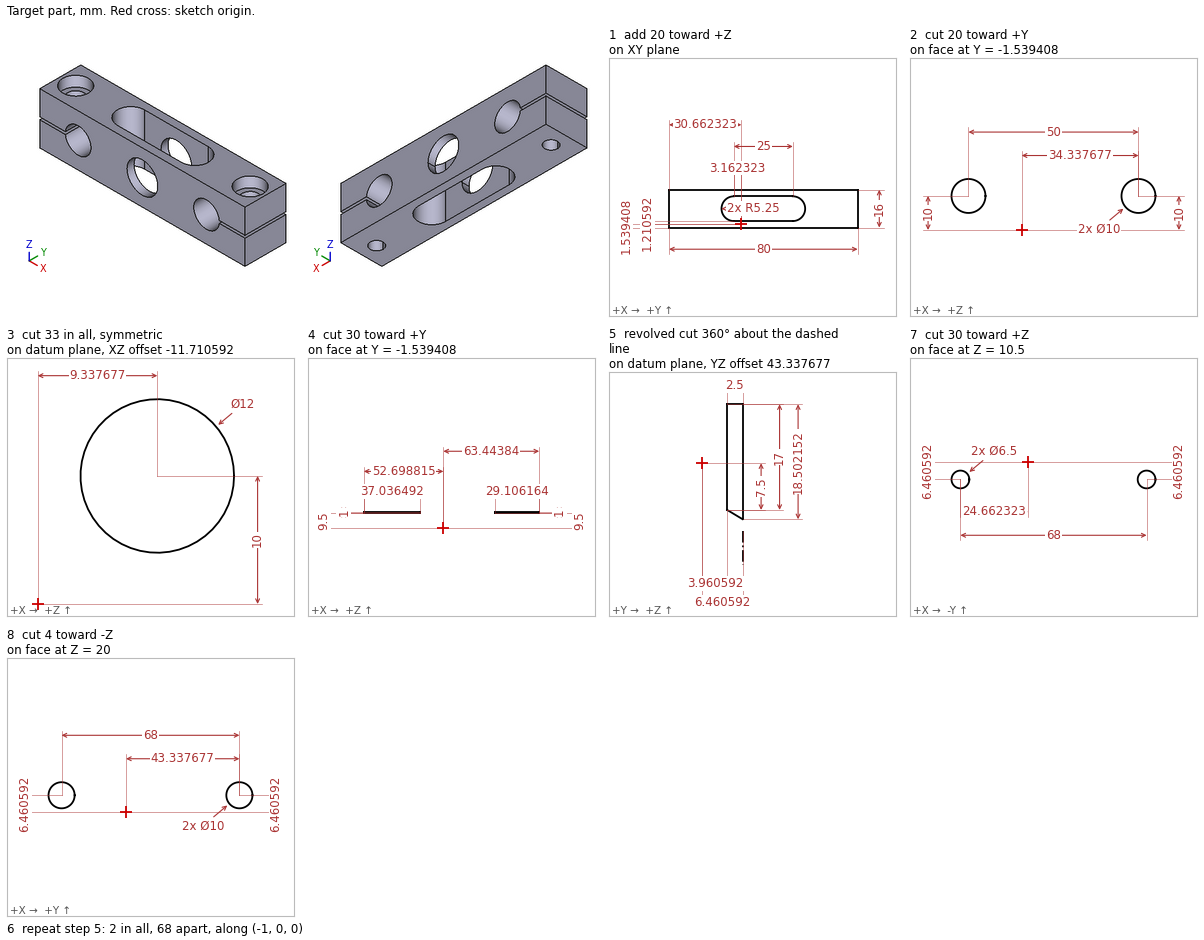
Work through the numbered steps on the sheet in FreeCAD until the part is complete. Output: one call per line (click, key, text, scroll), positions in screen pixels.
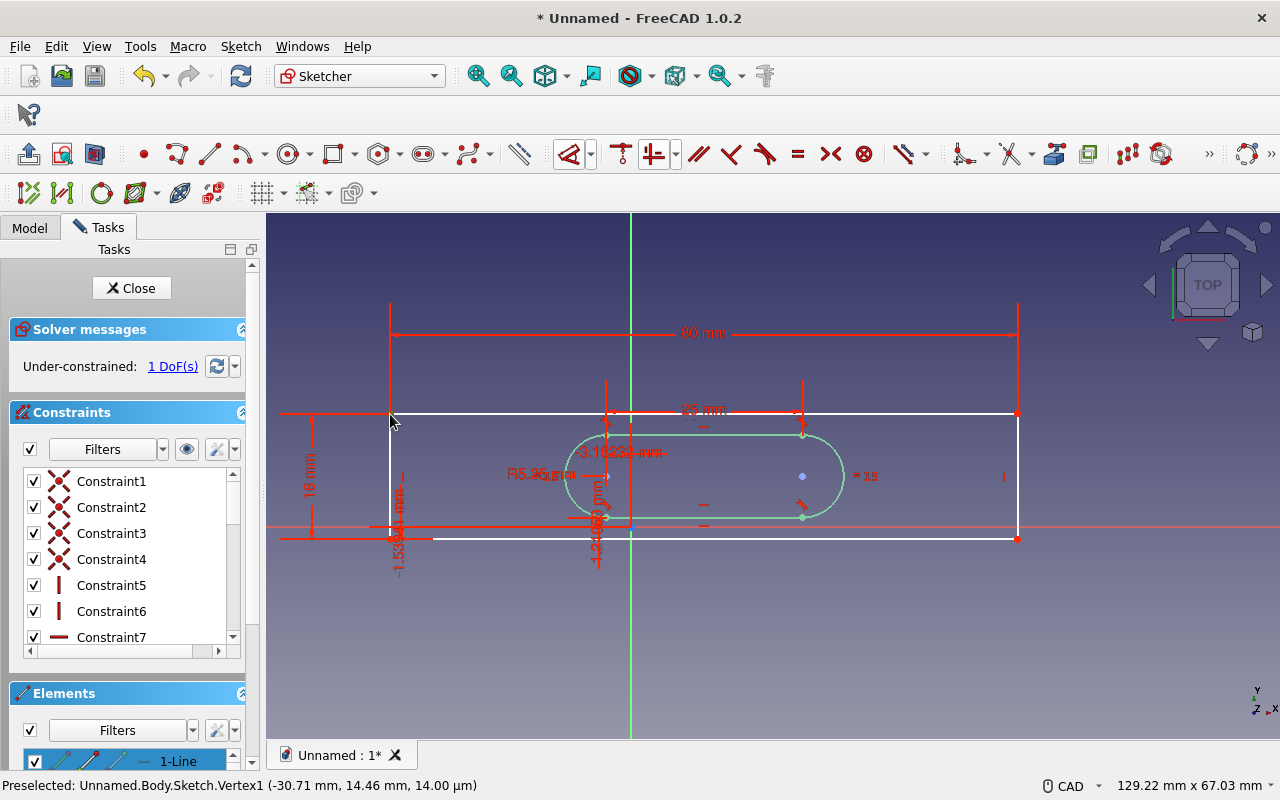
key(l)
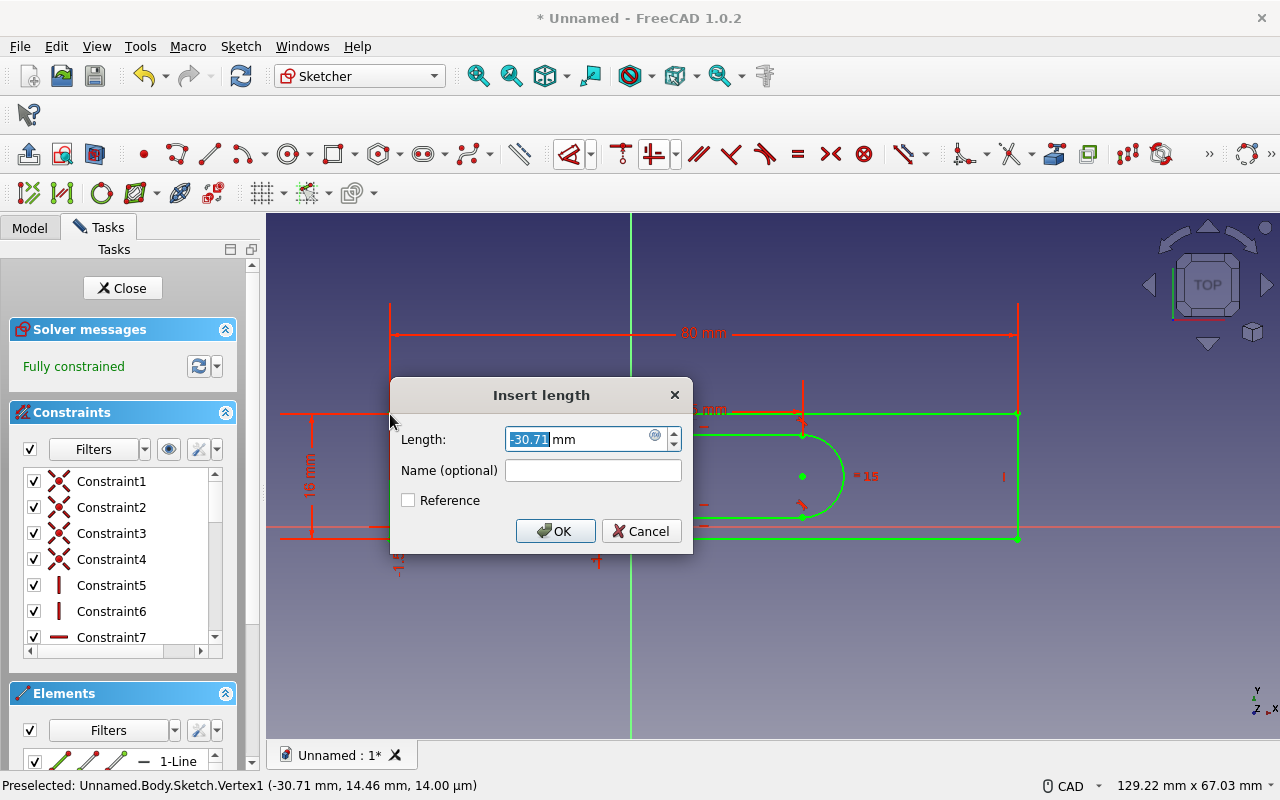
text(-30.662323)
key(Return)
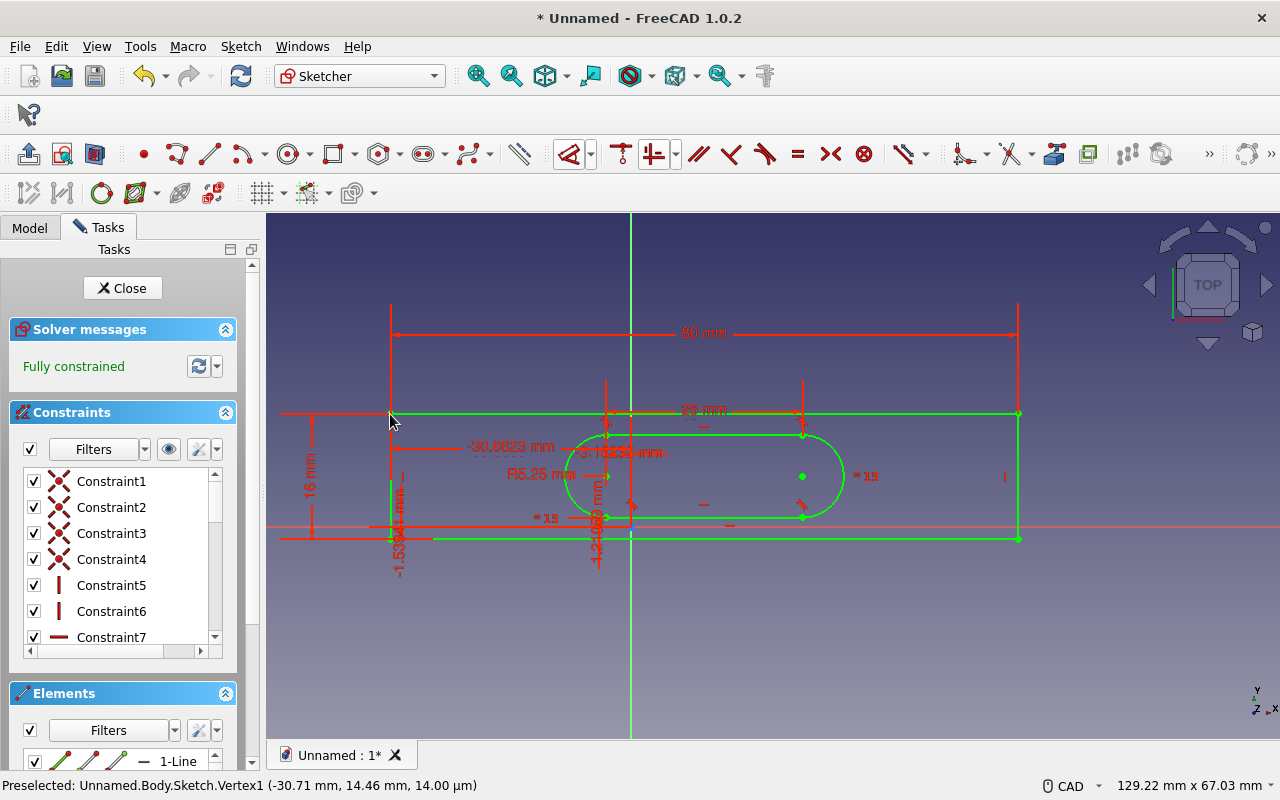
click(123, 288)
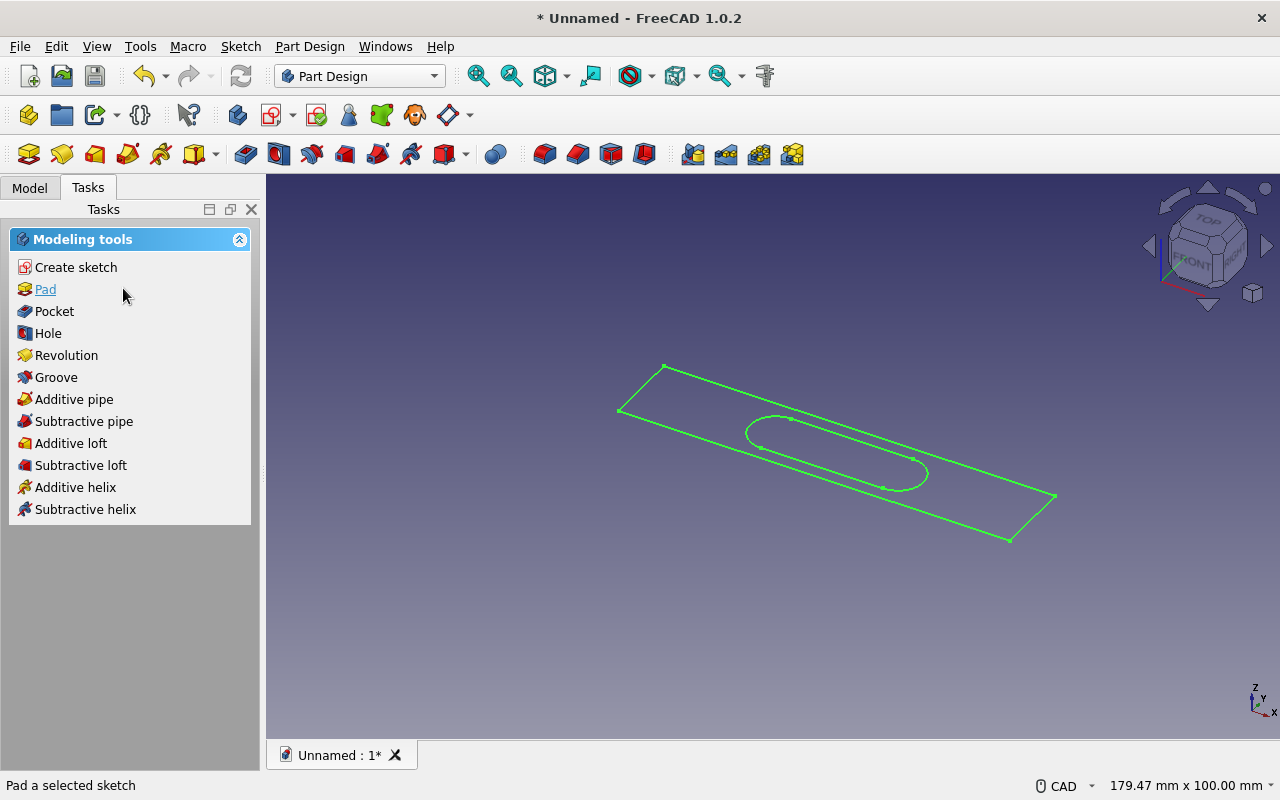
click(29, 154)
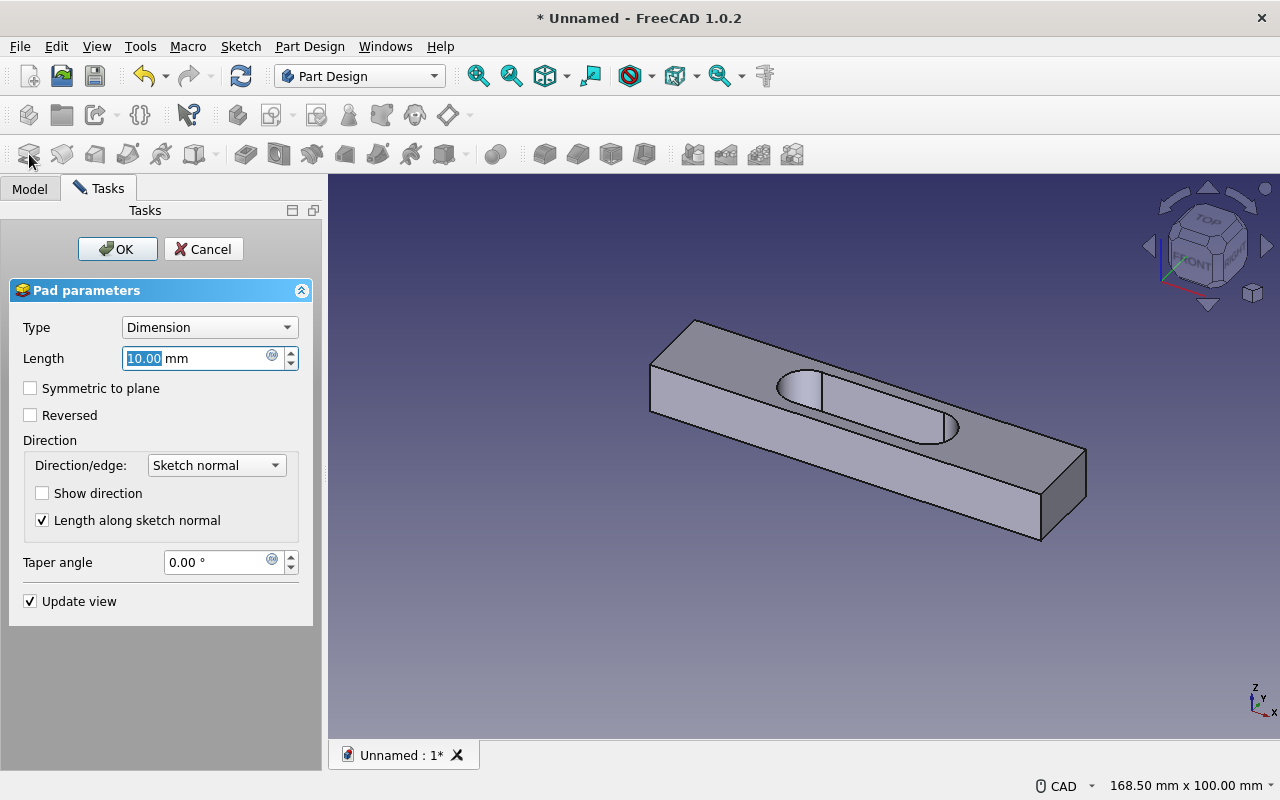
text(20)
key(Tab)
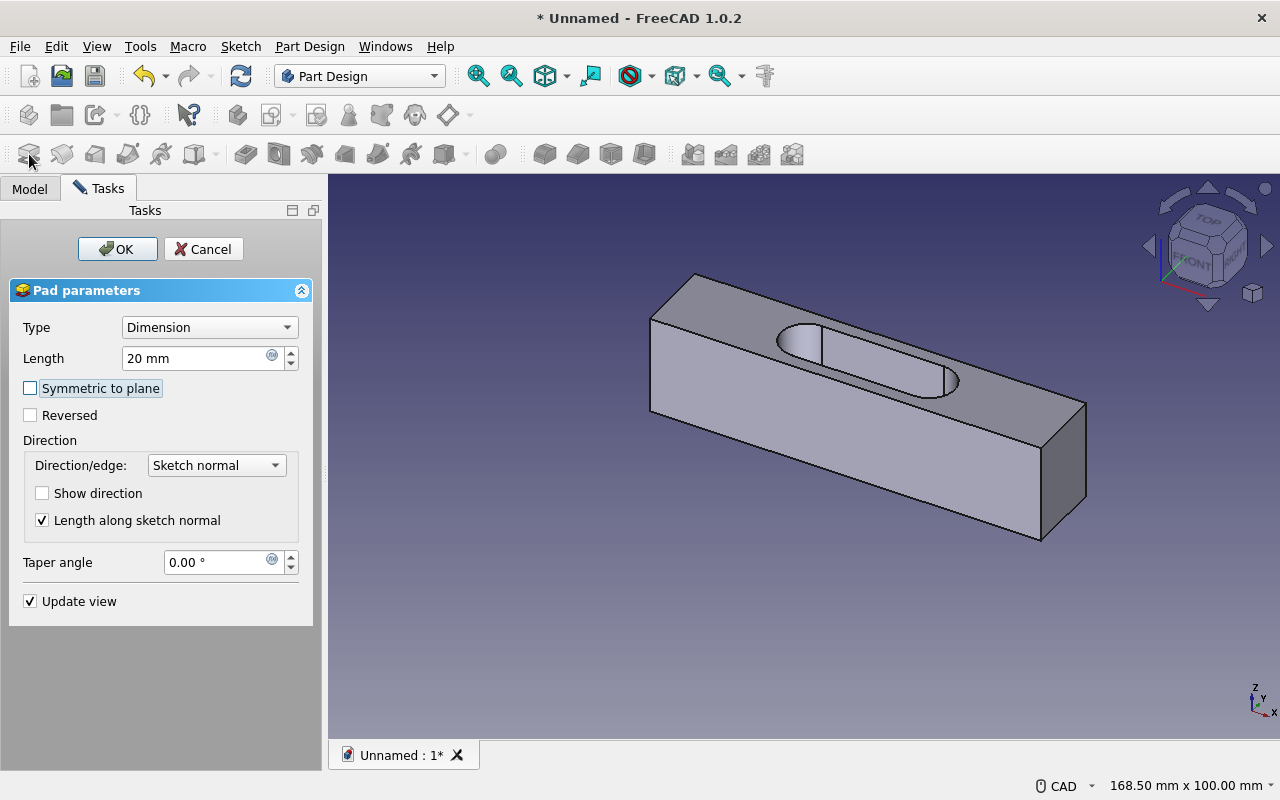
click(118, 249)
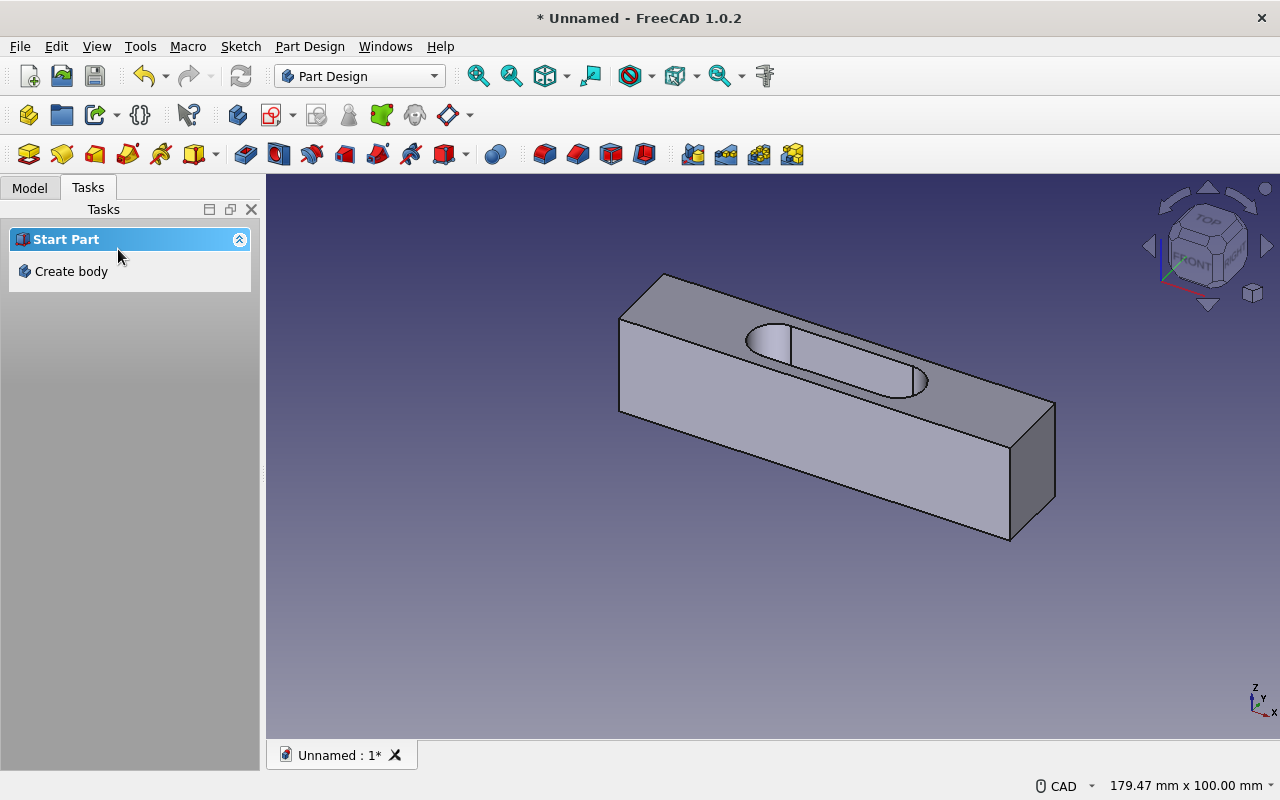
click(926, 466)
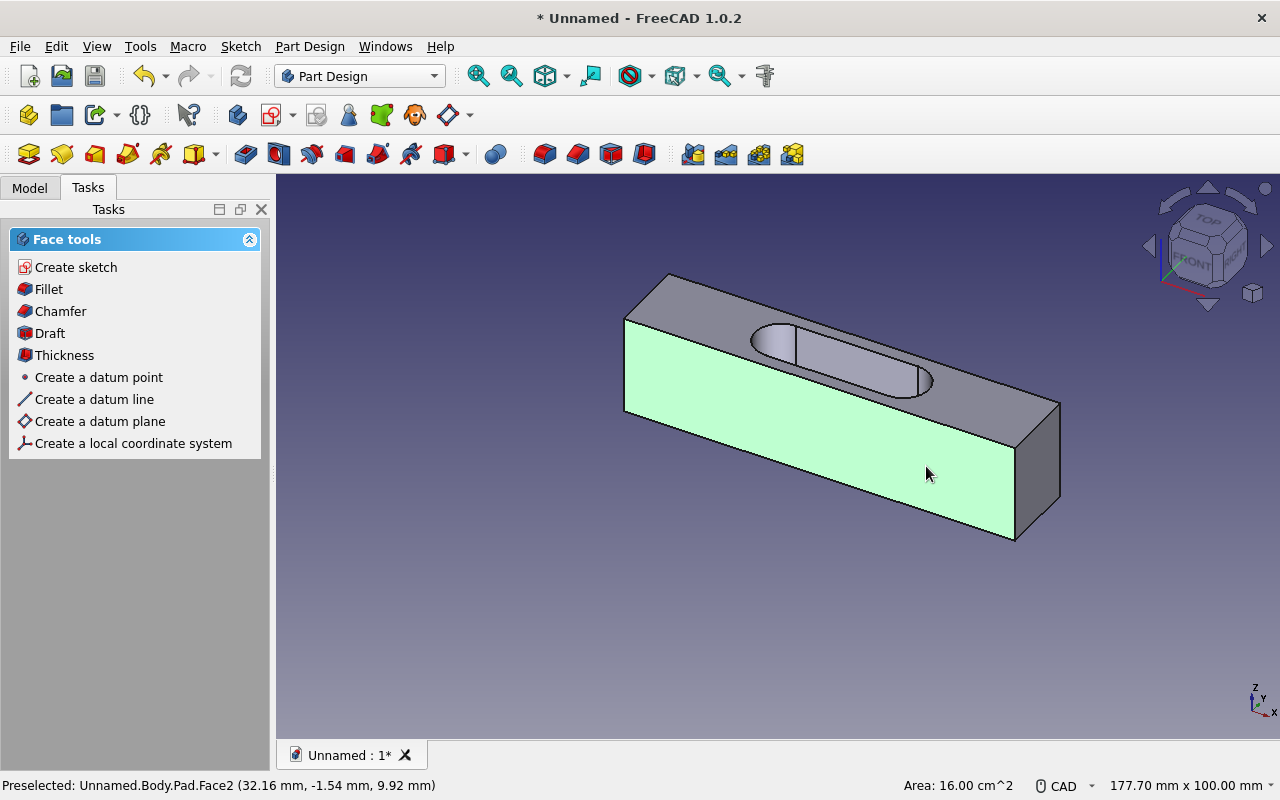
click(270, 116)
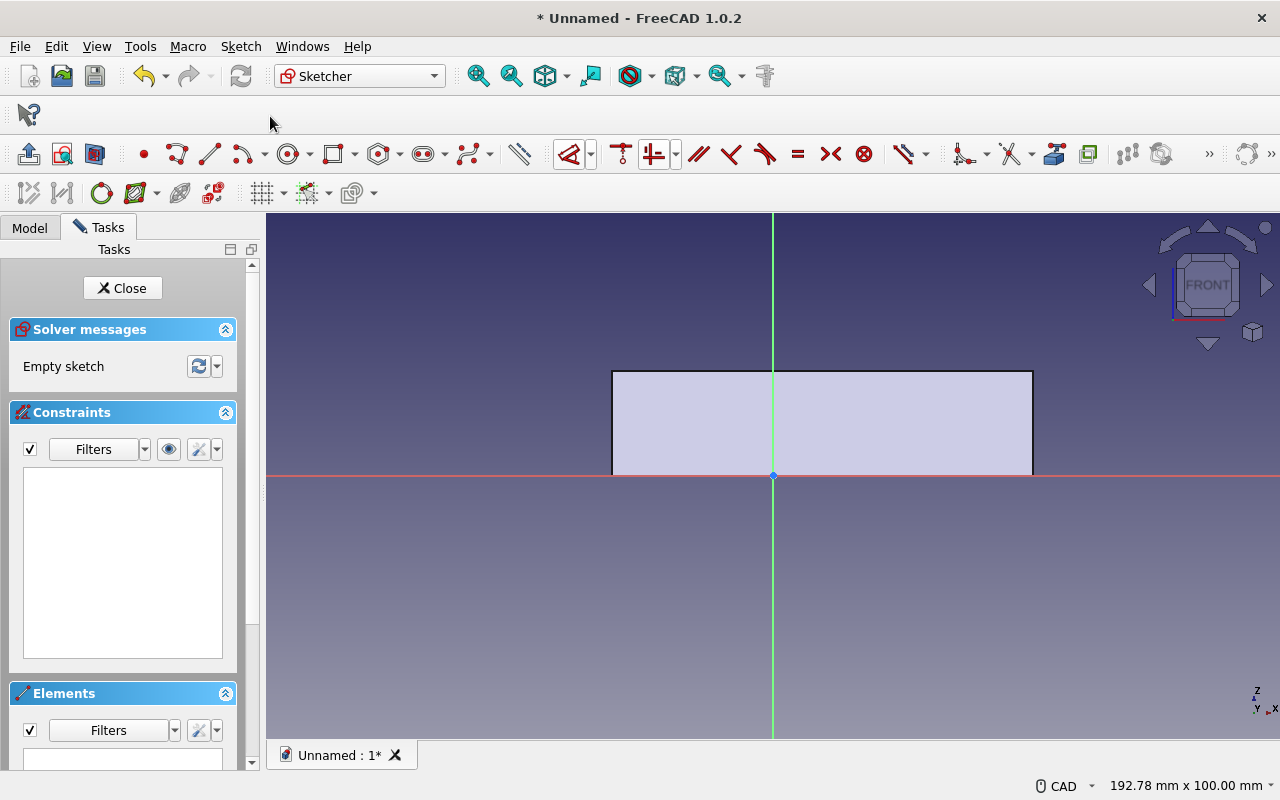
scroll(965, 389, up, 3)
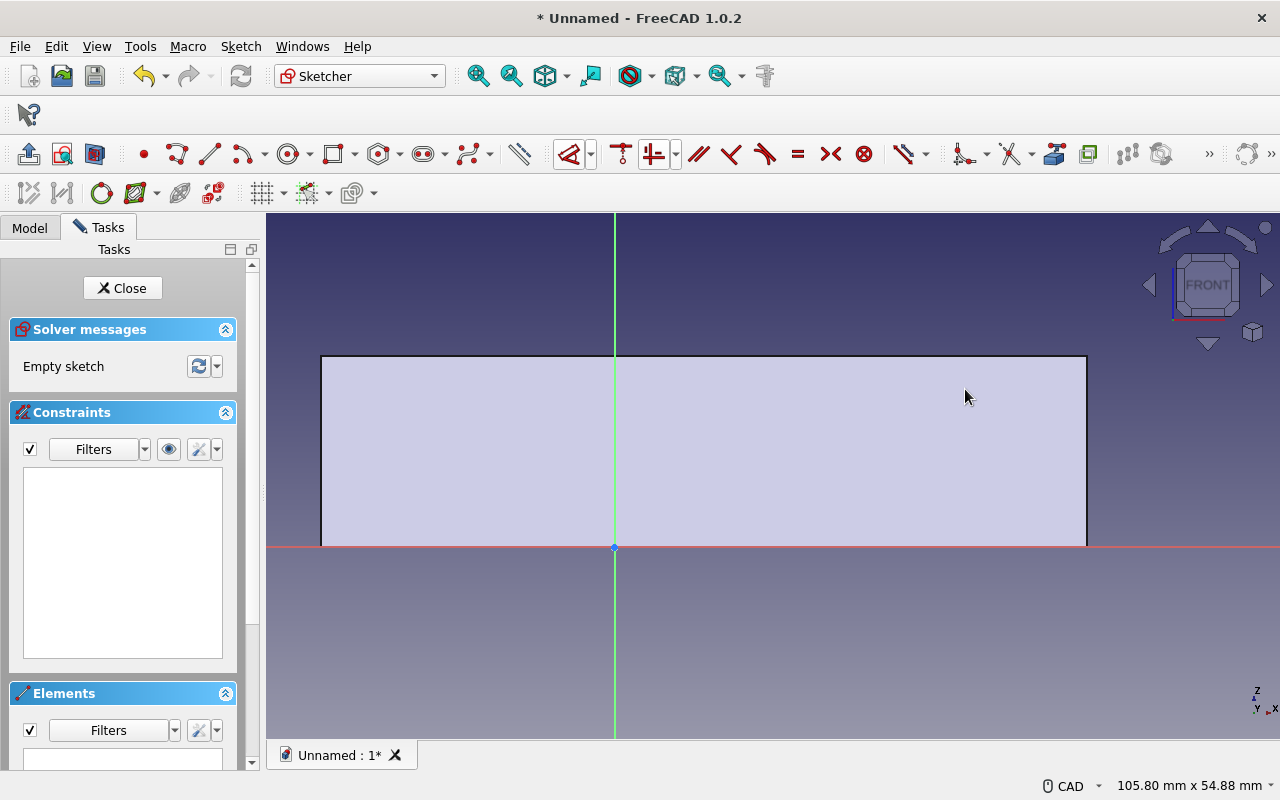
key(g)
key(c)